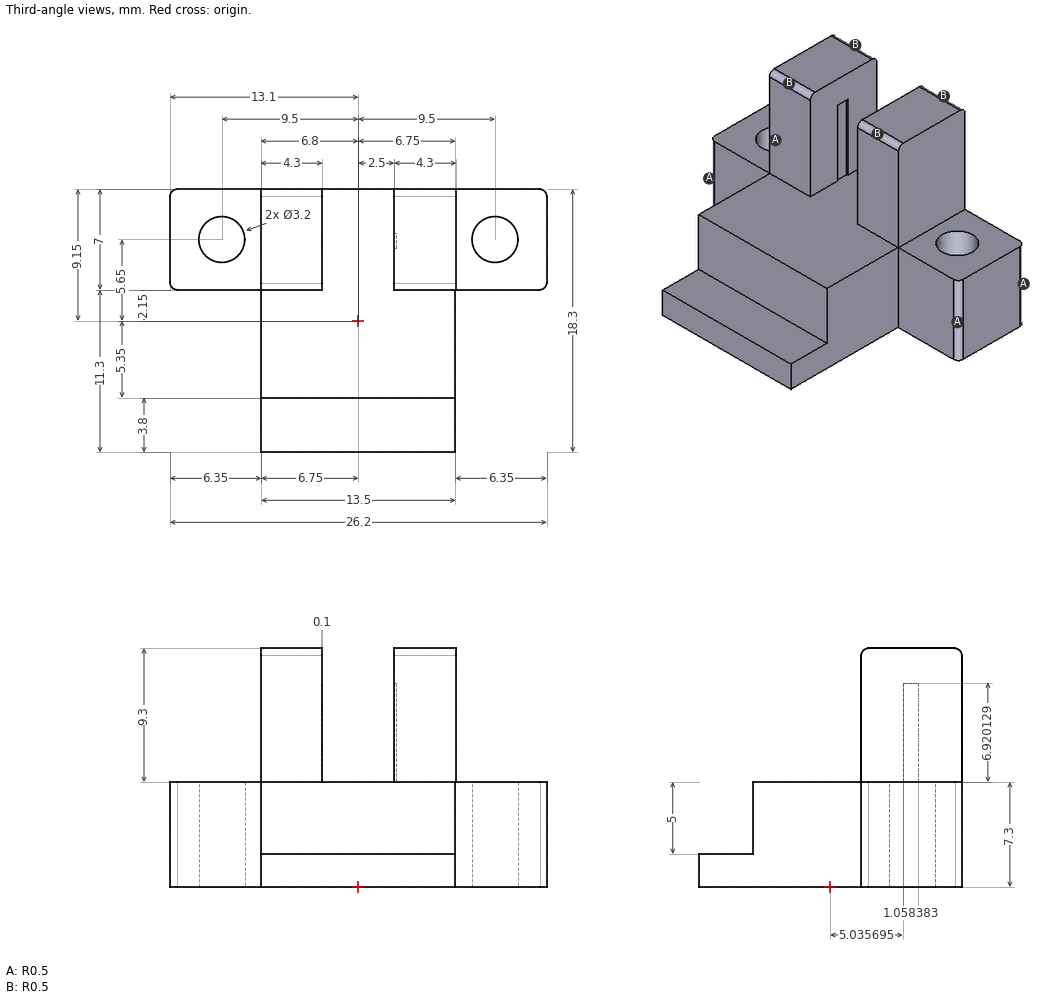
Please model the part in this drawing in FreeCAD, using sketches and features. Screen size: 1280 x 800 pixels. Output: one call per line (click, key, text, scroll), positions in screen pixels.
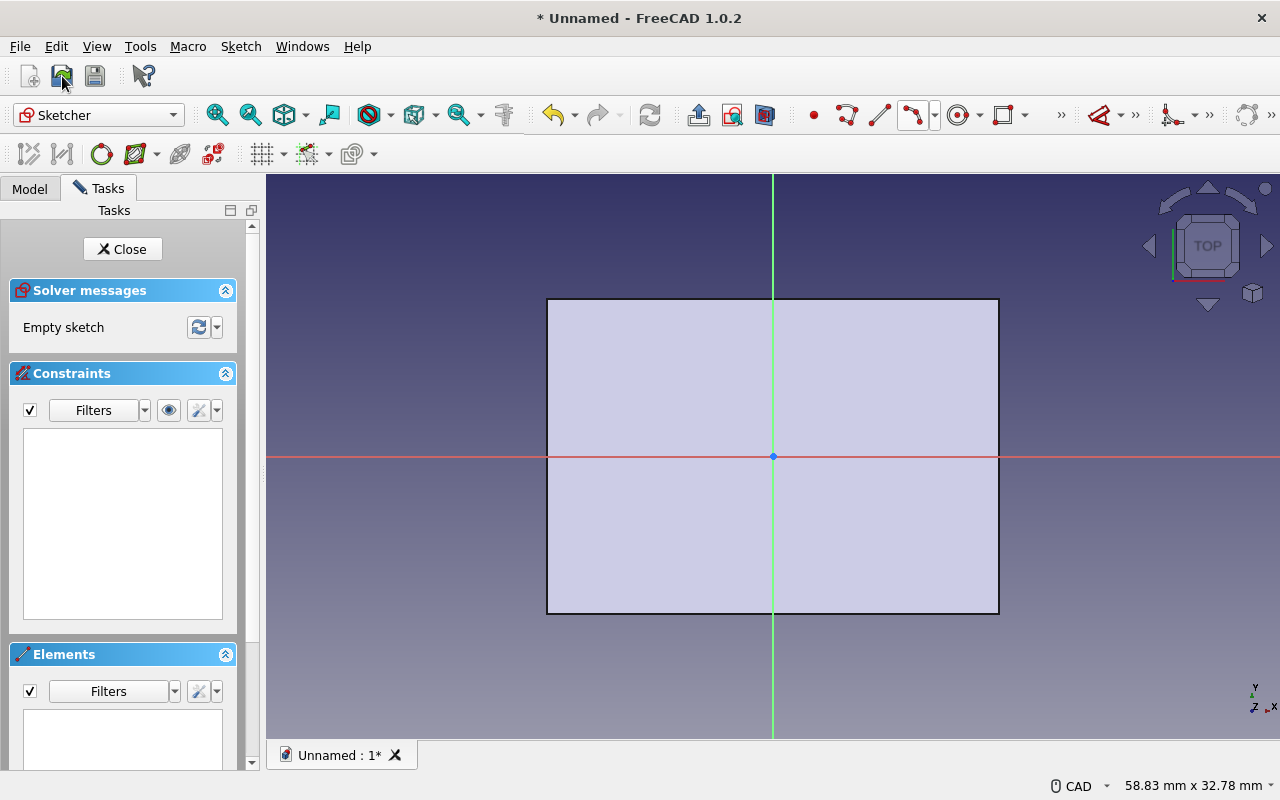
click(1002, 116)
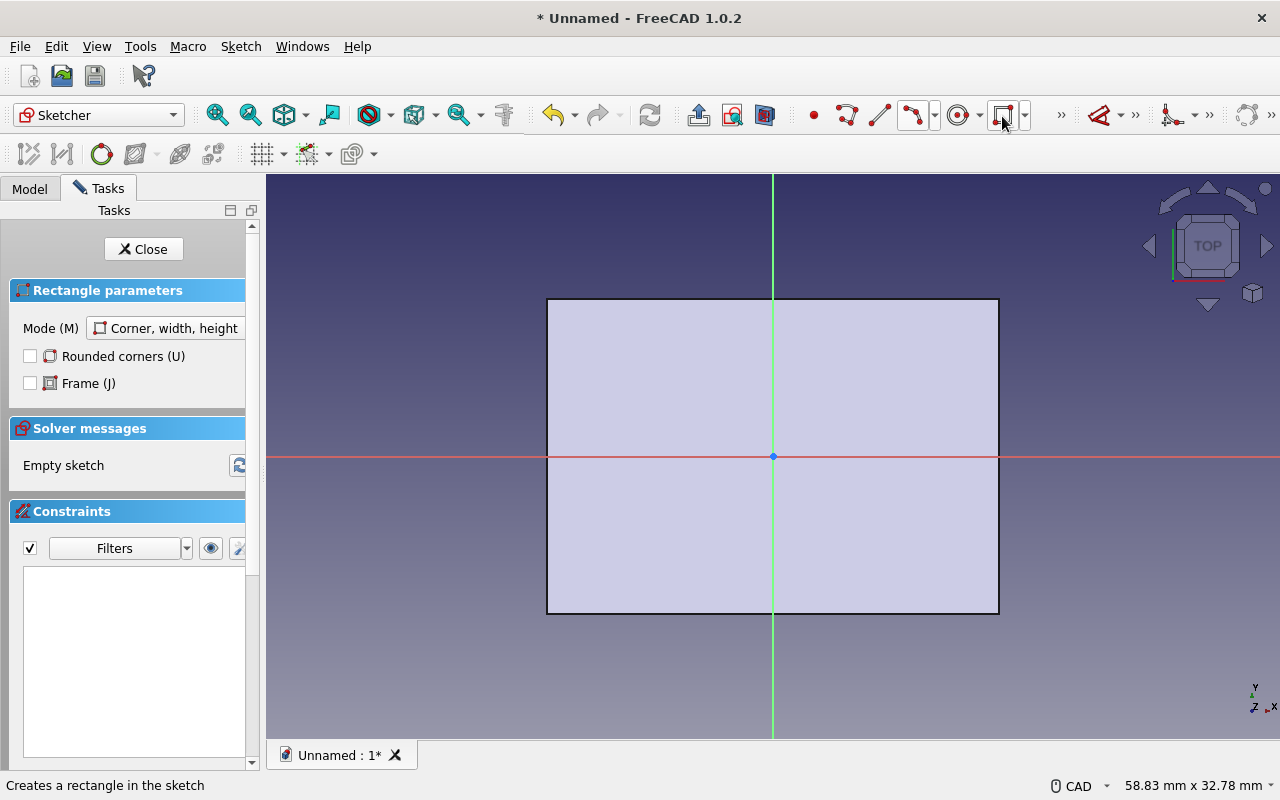
click(547, 419)
click(657, 614)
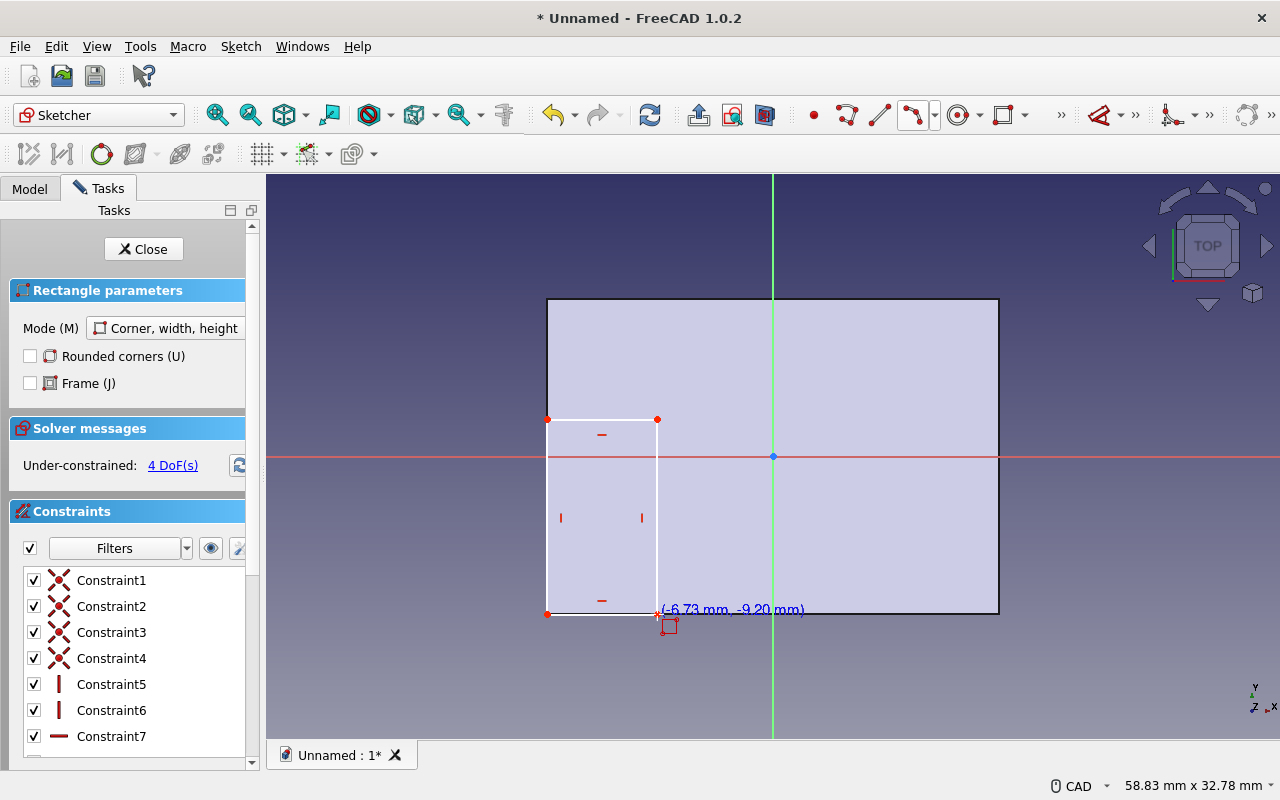
click(889, 419)
click(999, 614)
key(Escape)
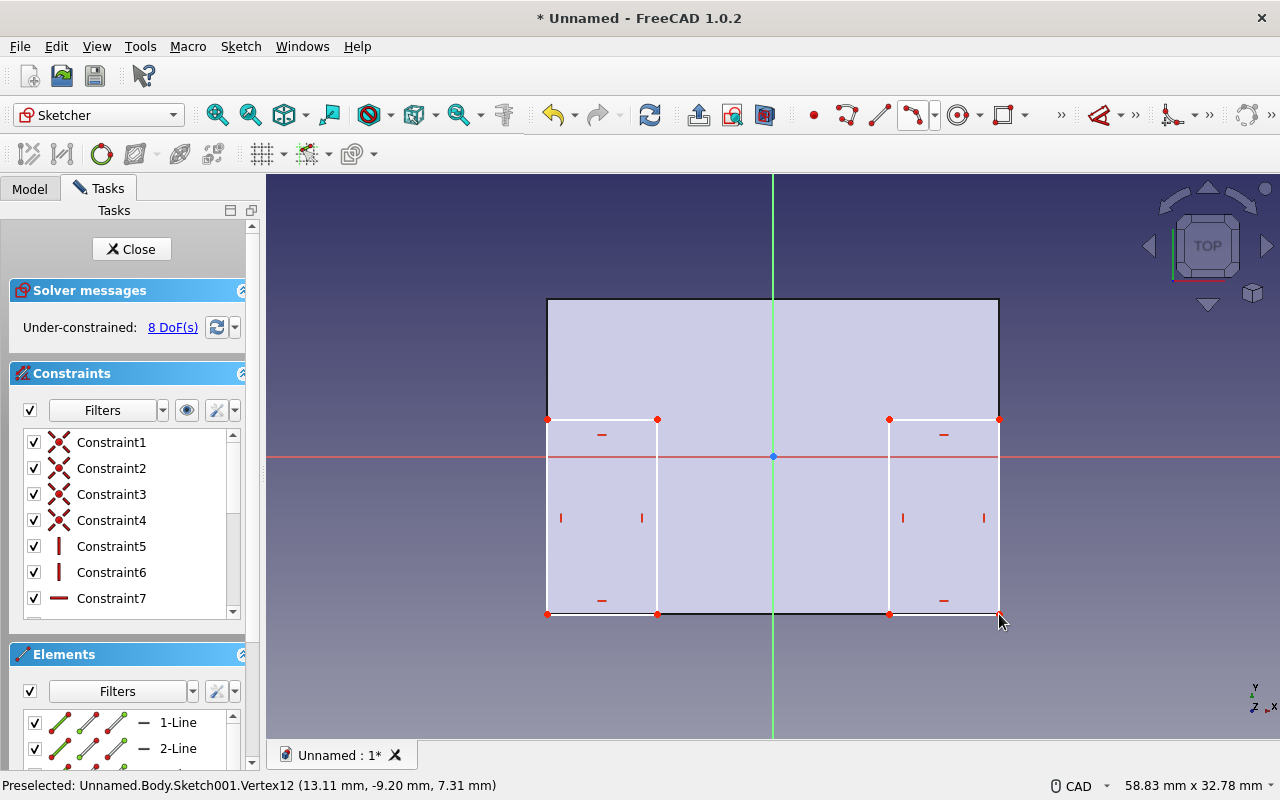
click(547, 478)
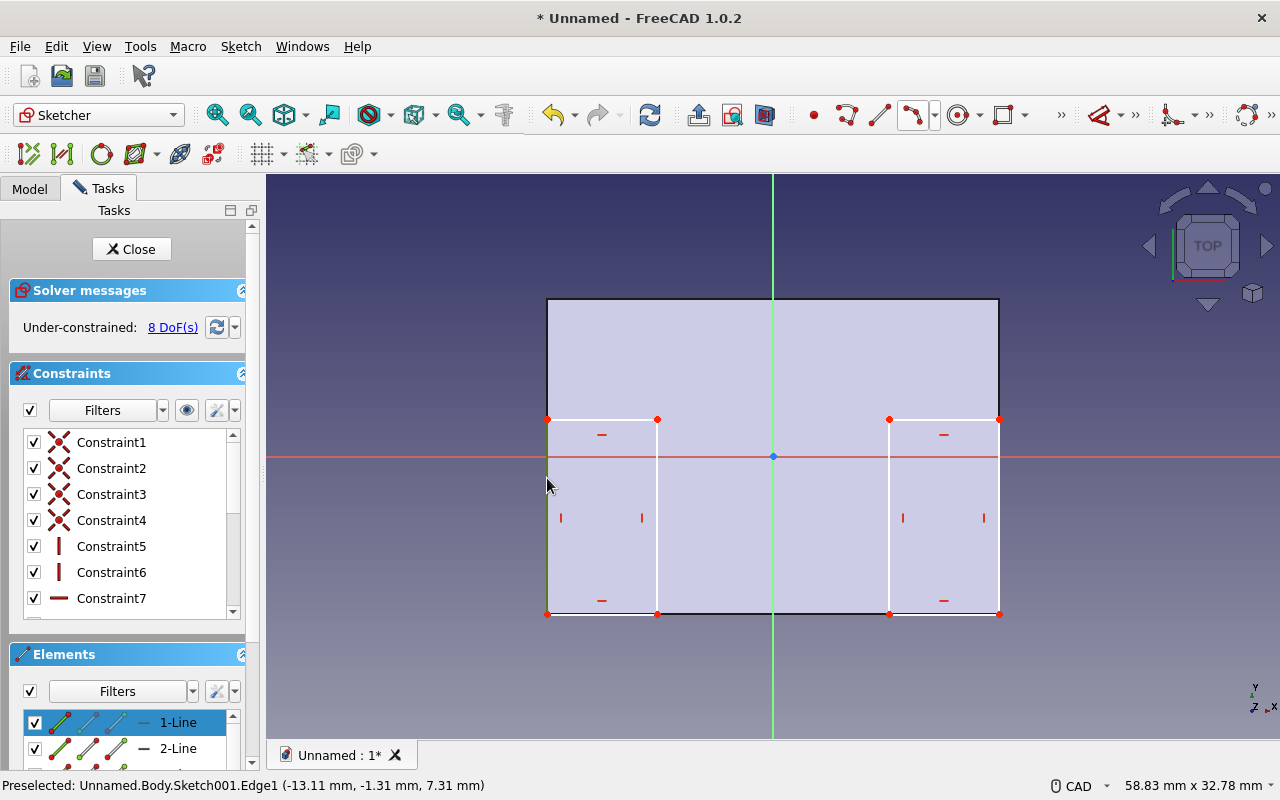
key(i)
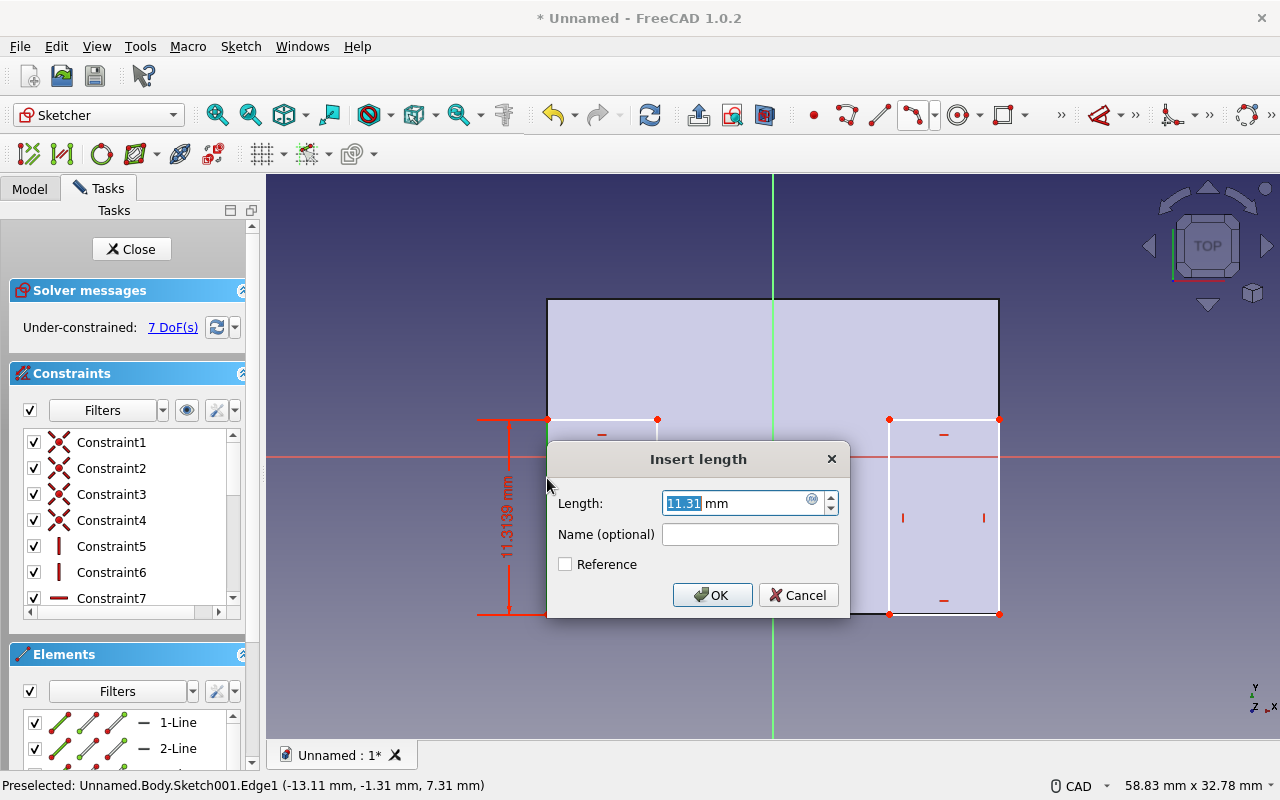
text(11.3)
key(Return)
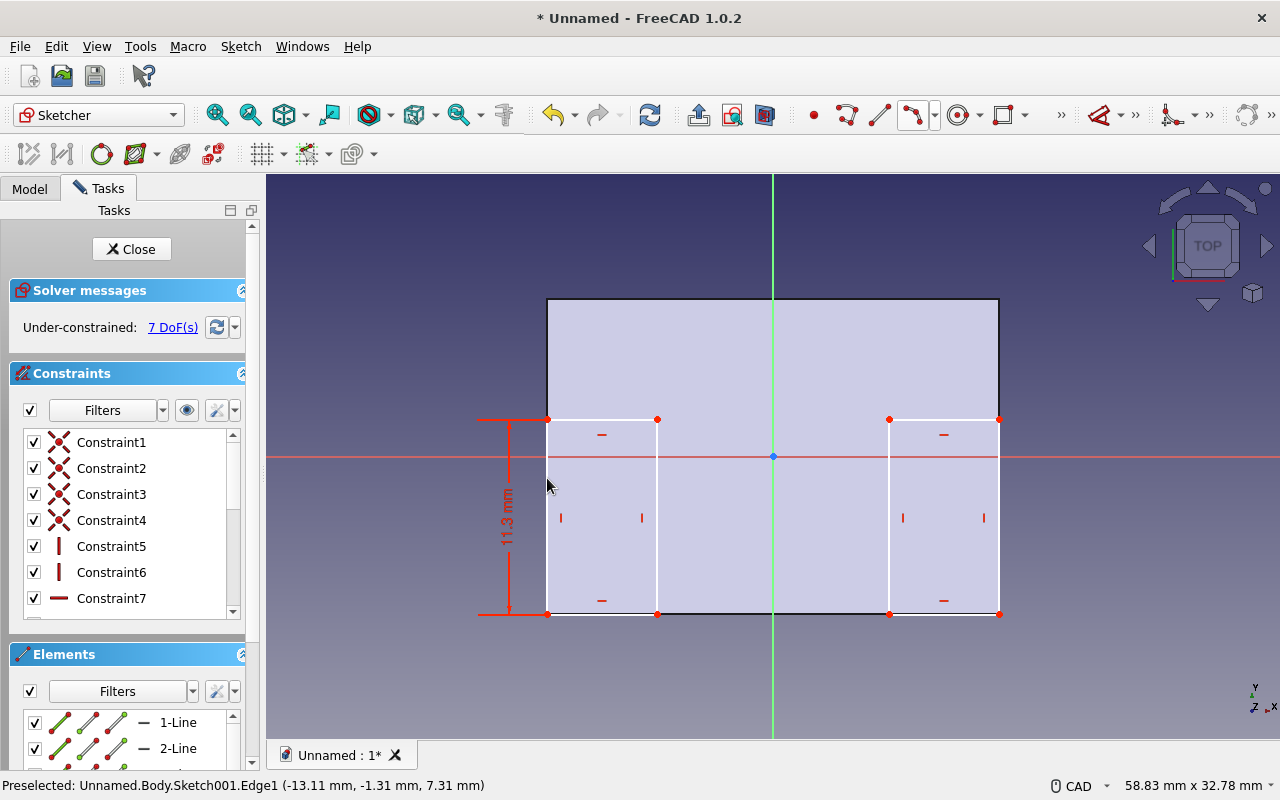
click(580, 615)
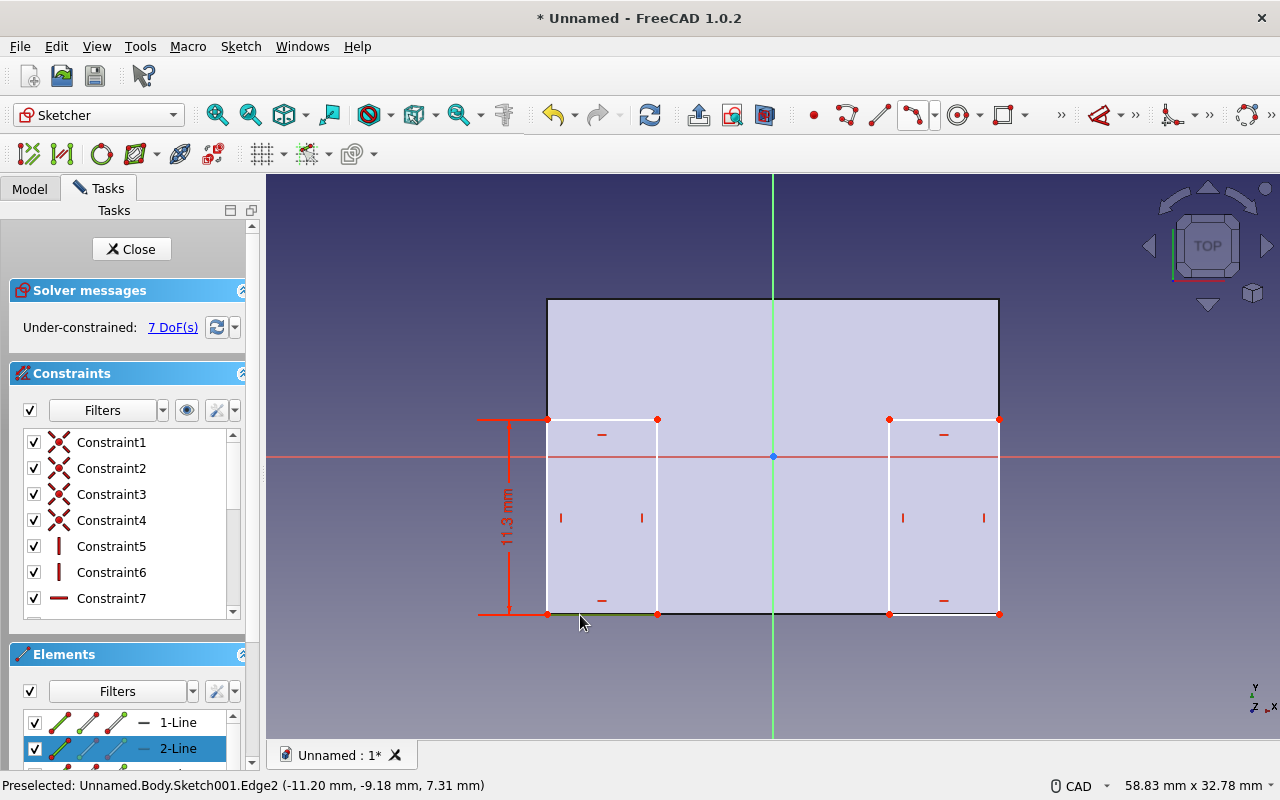
key(l)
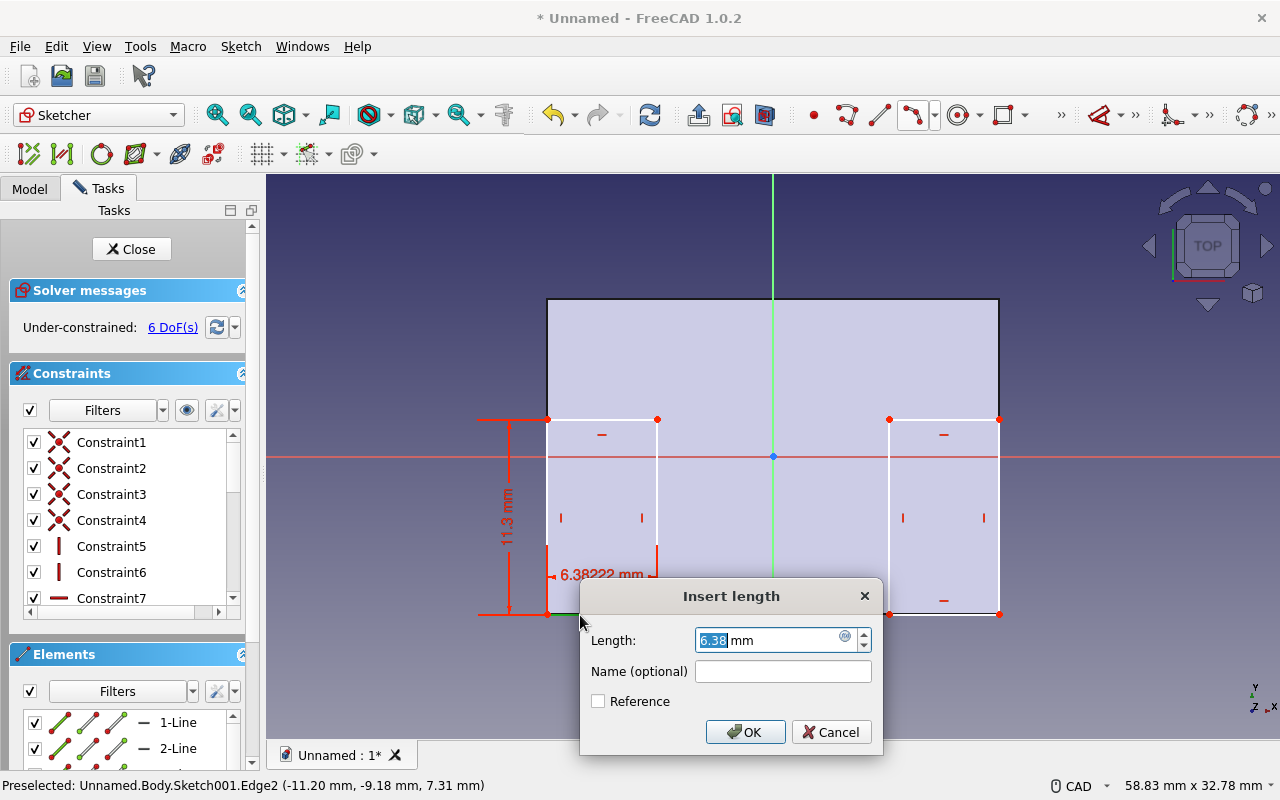
text(6.35)
key(Return)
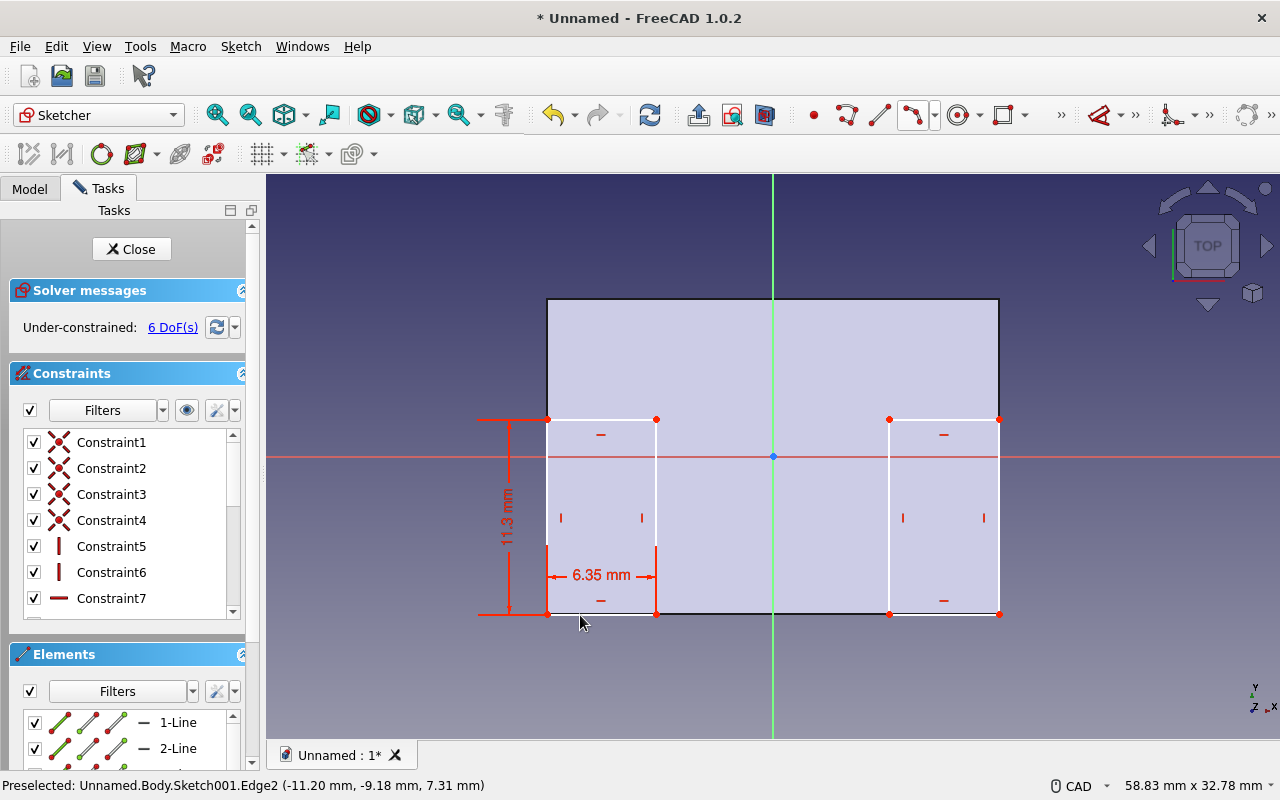
click(889, 478)